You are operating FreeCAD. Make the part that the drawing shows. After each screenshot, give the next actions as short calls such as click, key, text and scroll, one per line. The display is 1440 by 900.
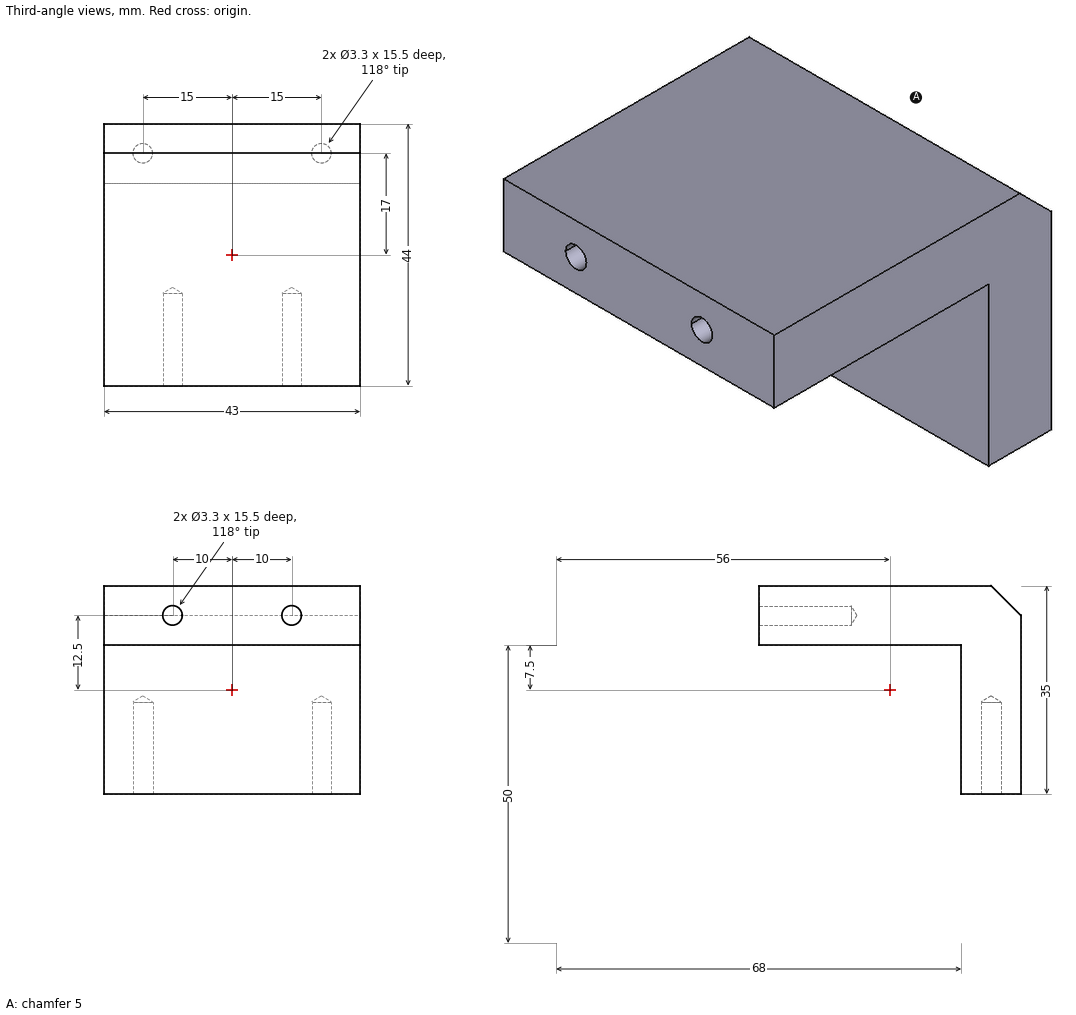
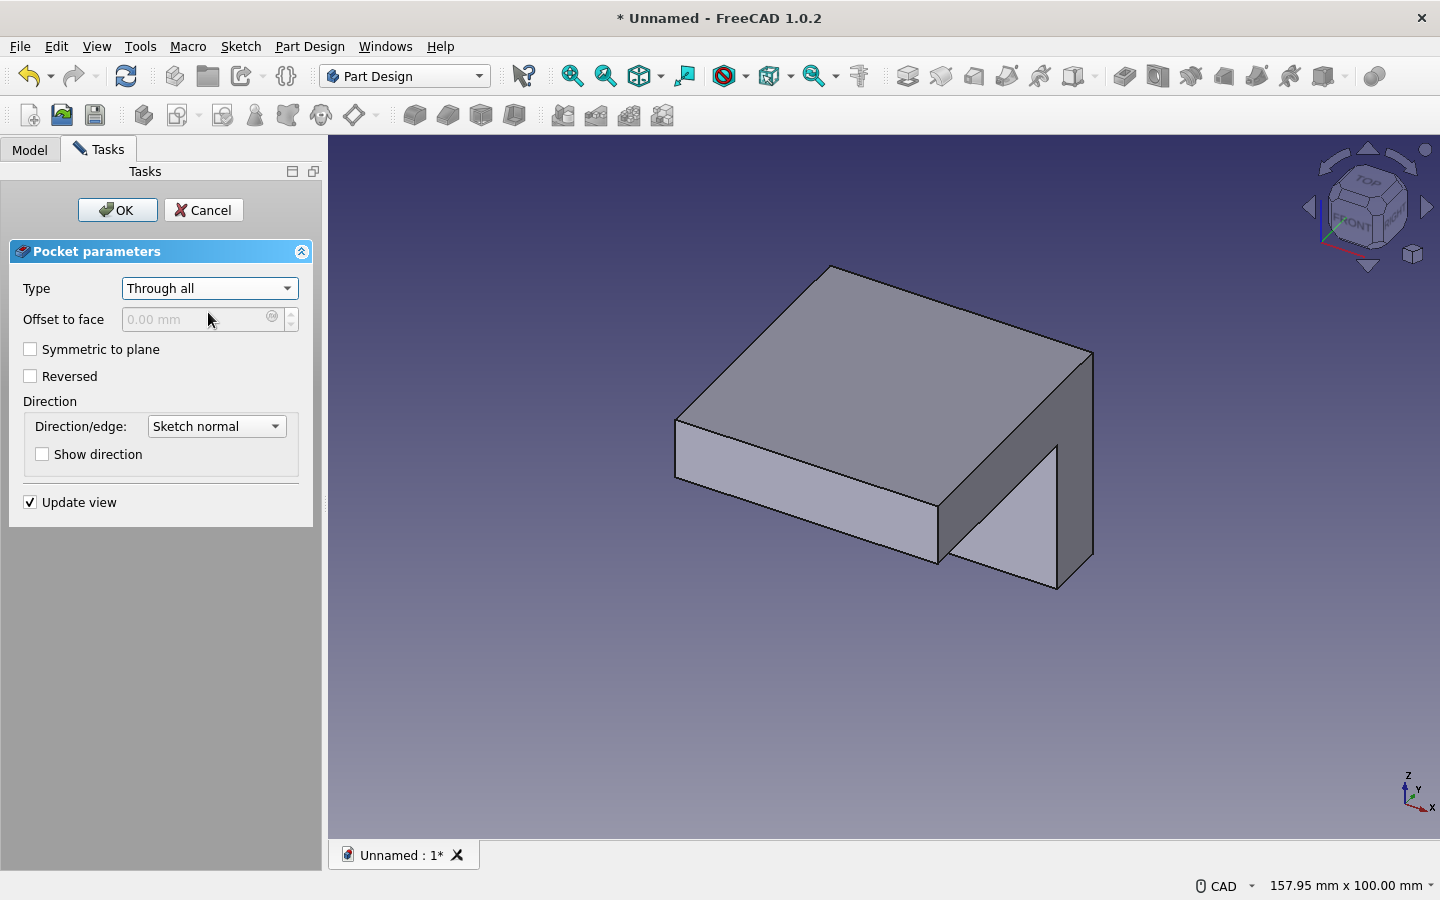
click(118, 210)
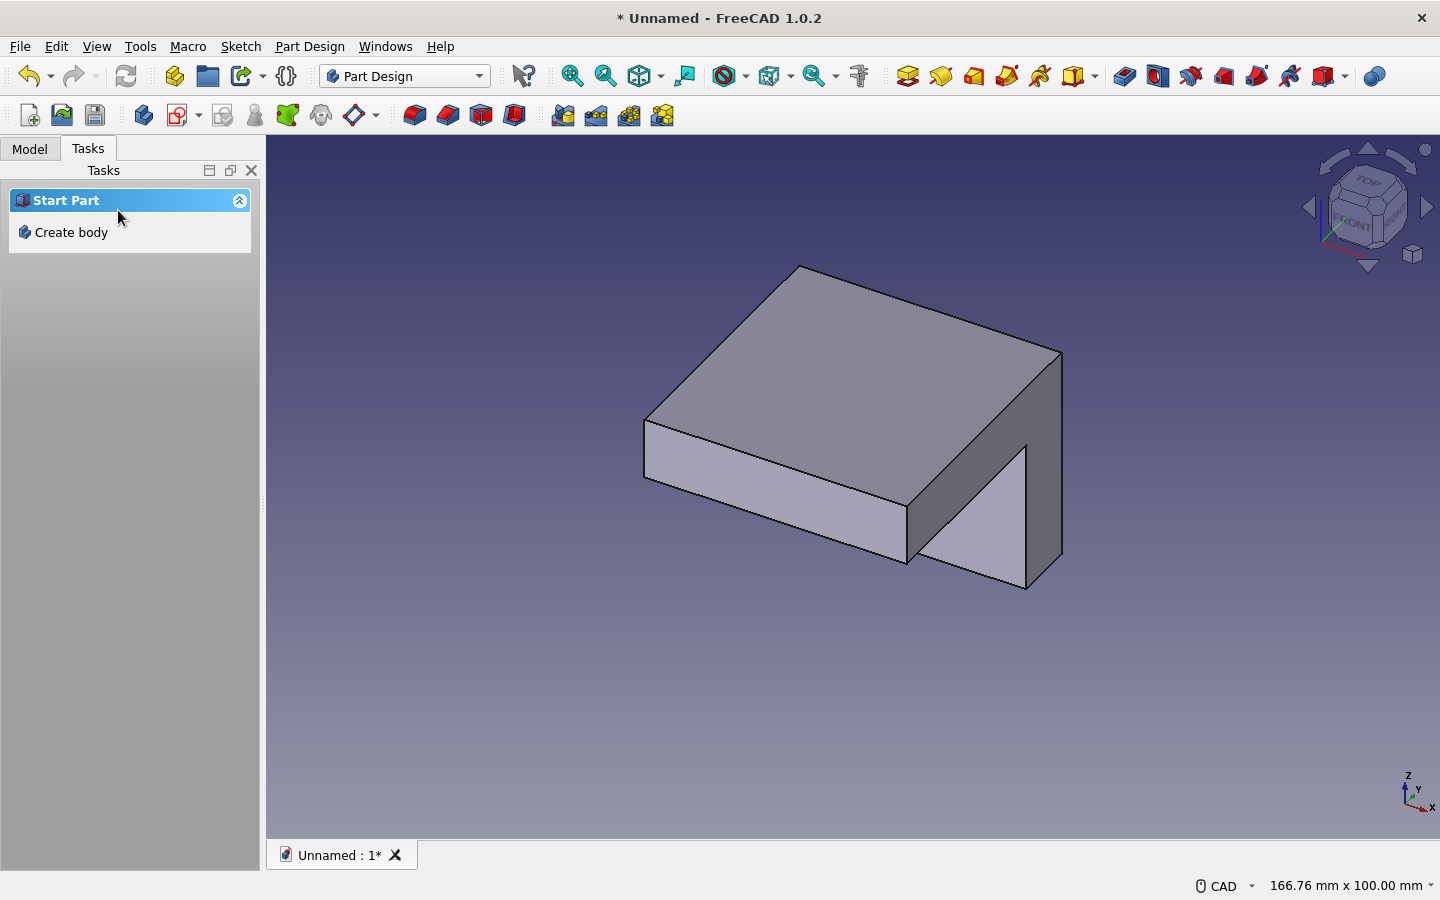
key(5)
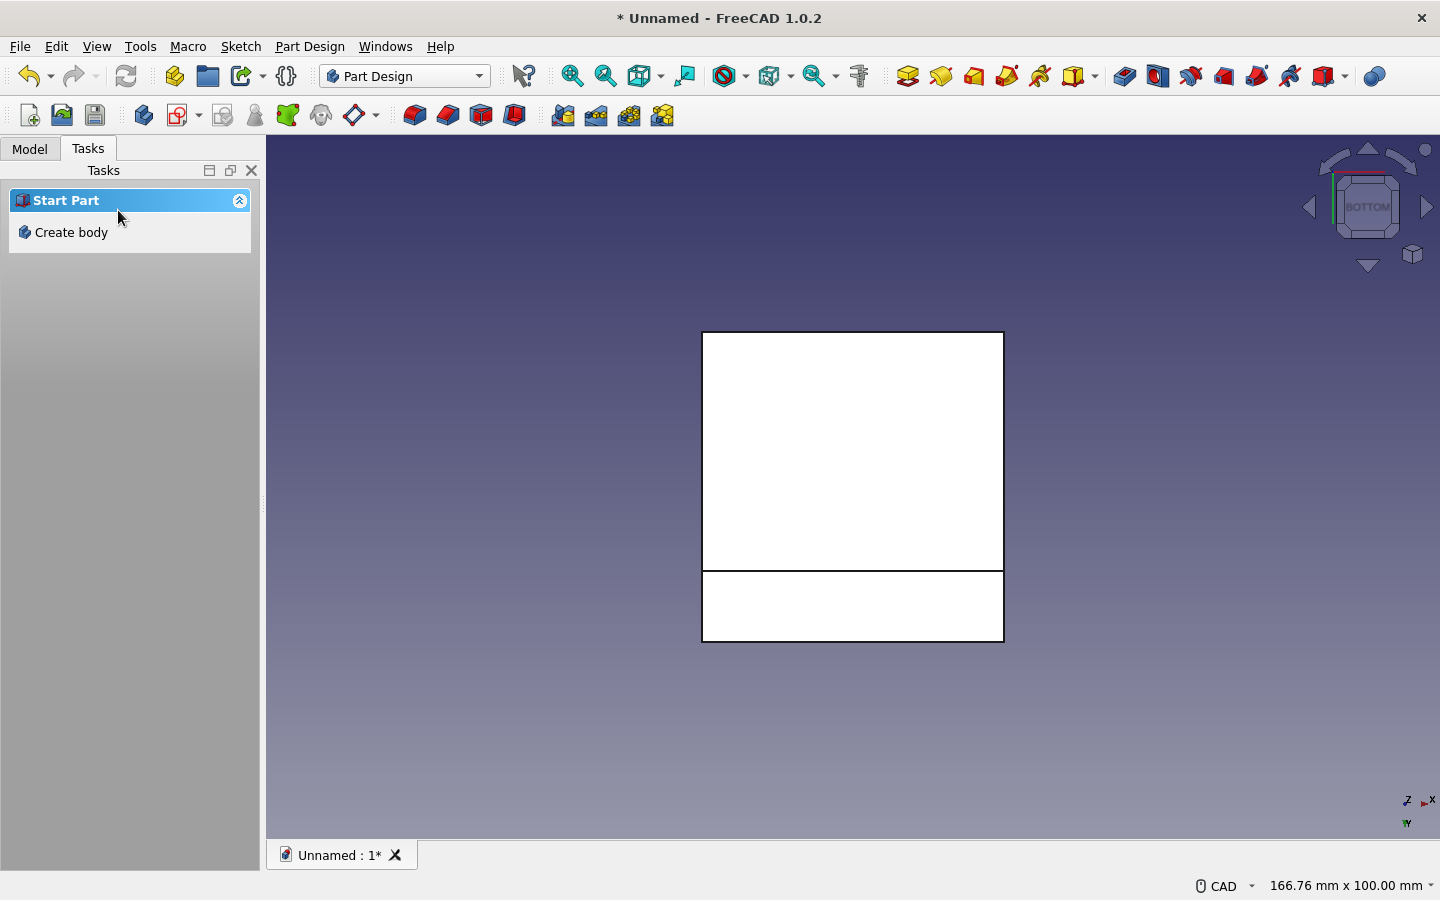
click(573, 76)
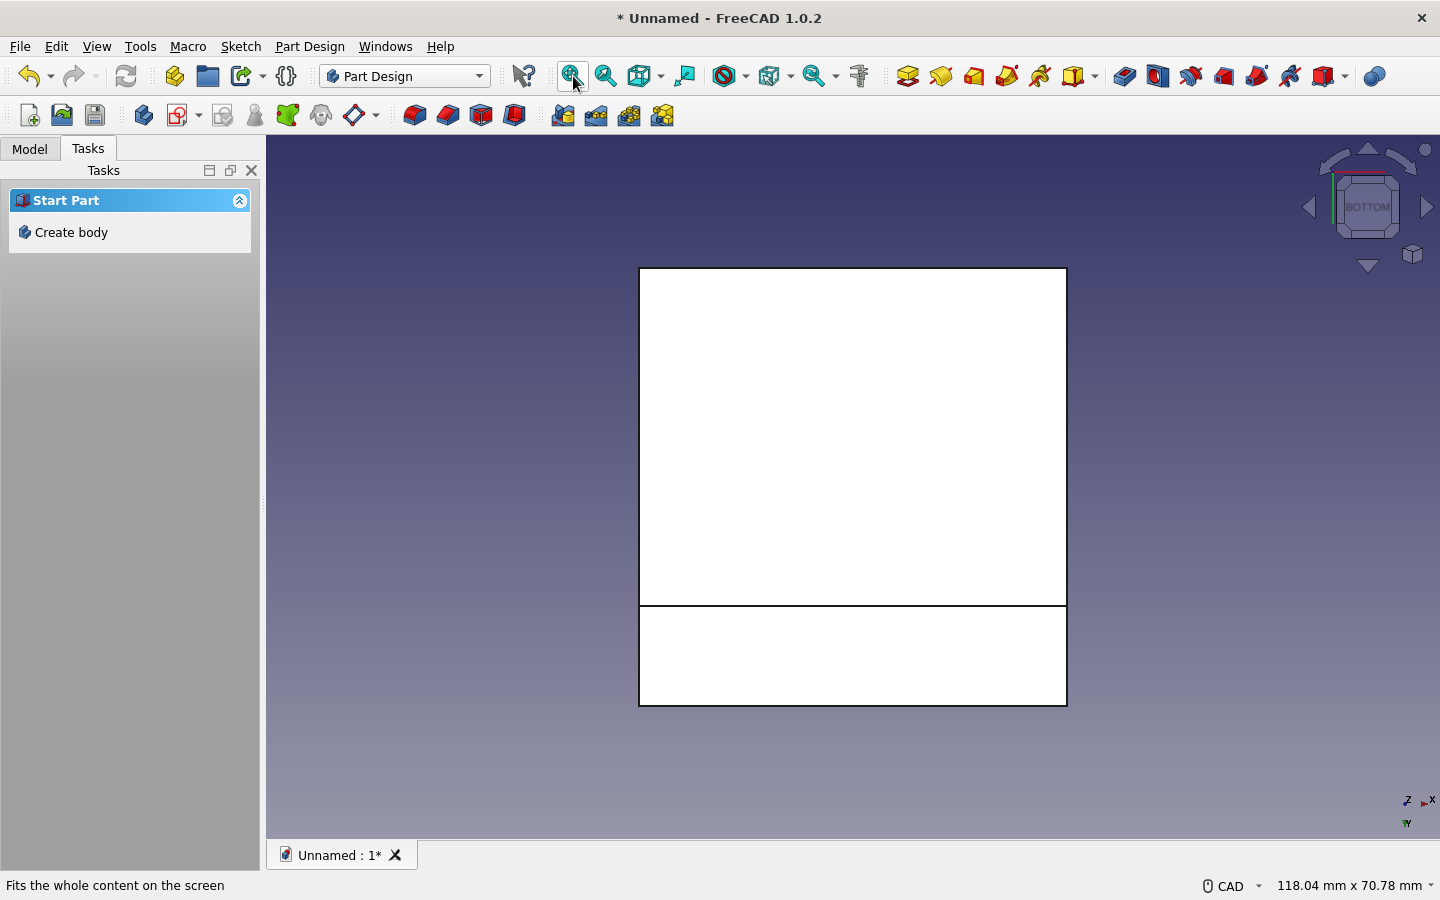
click(975, 655)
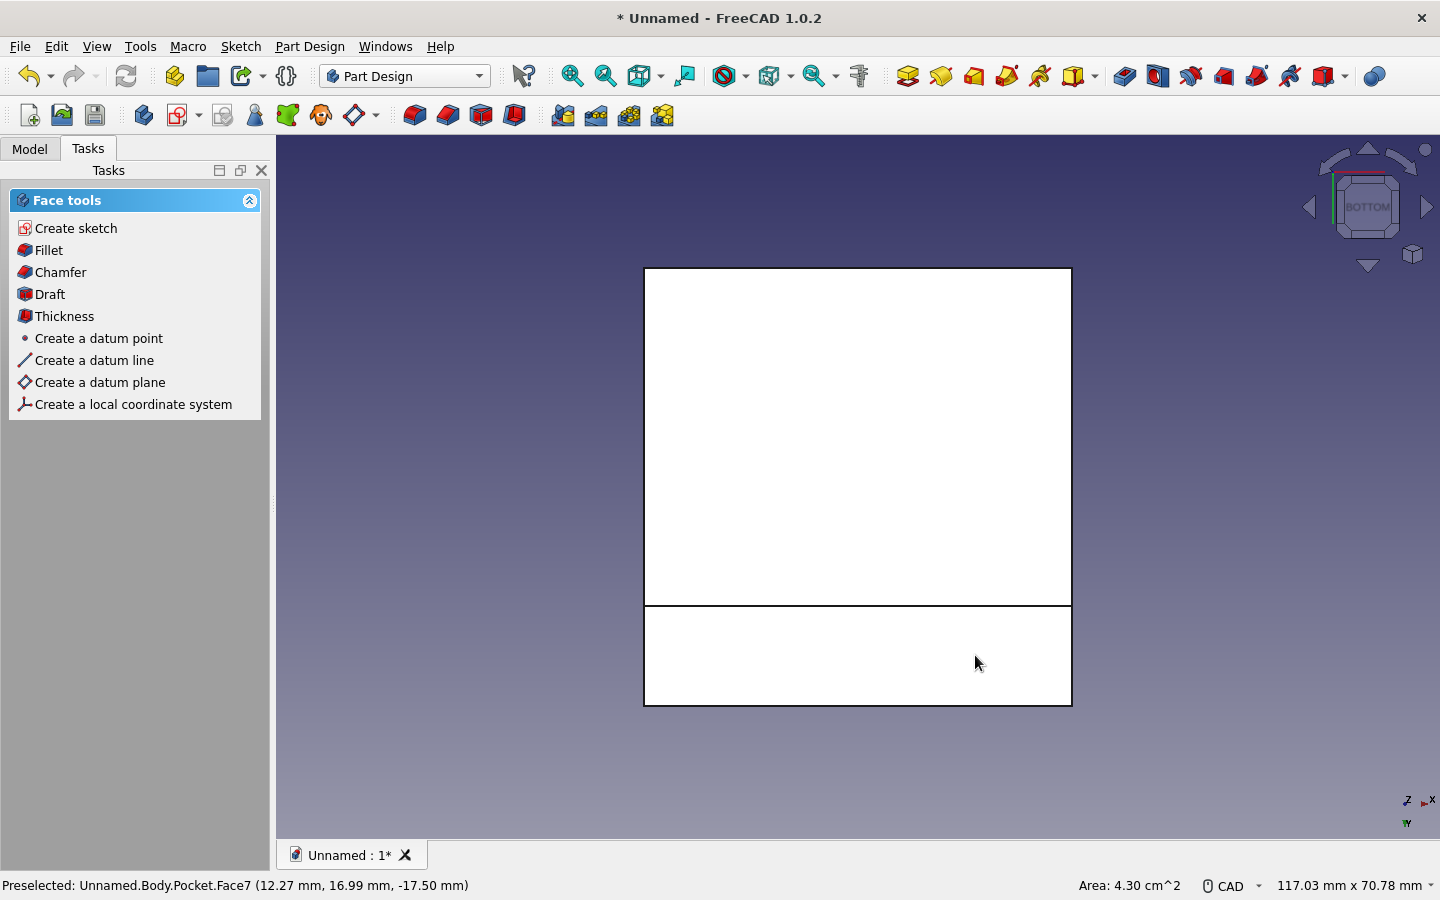
click(176, 116)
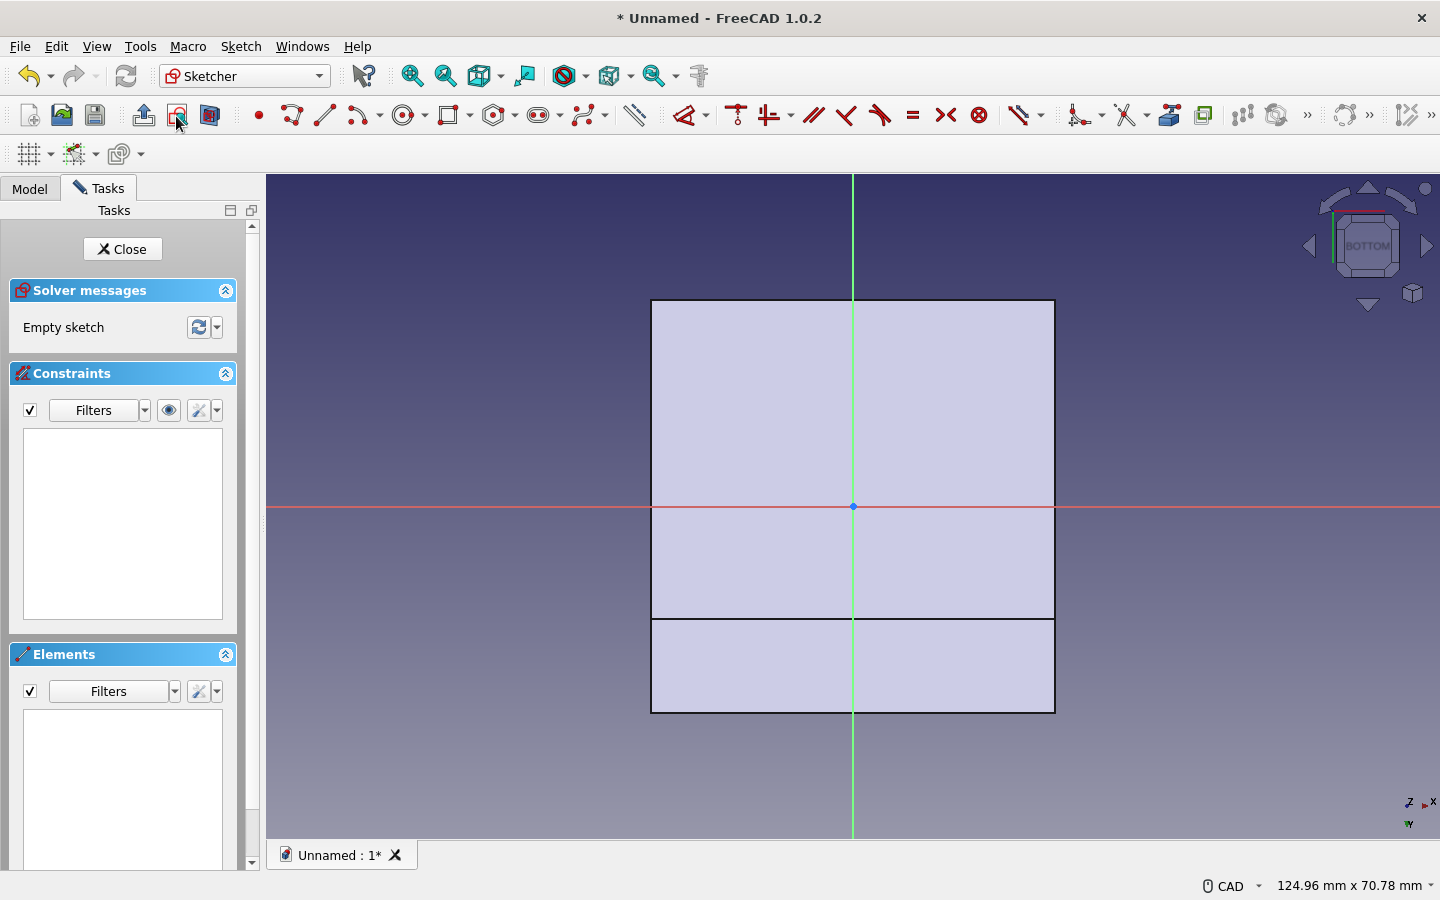
scroll(909, 666, up, 4)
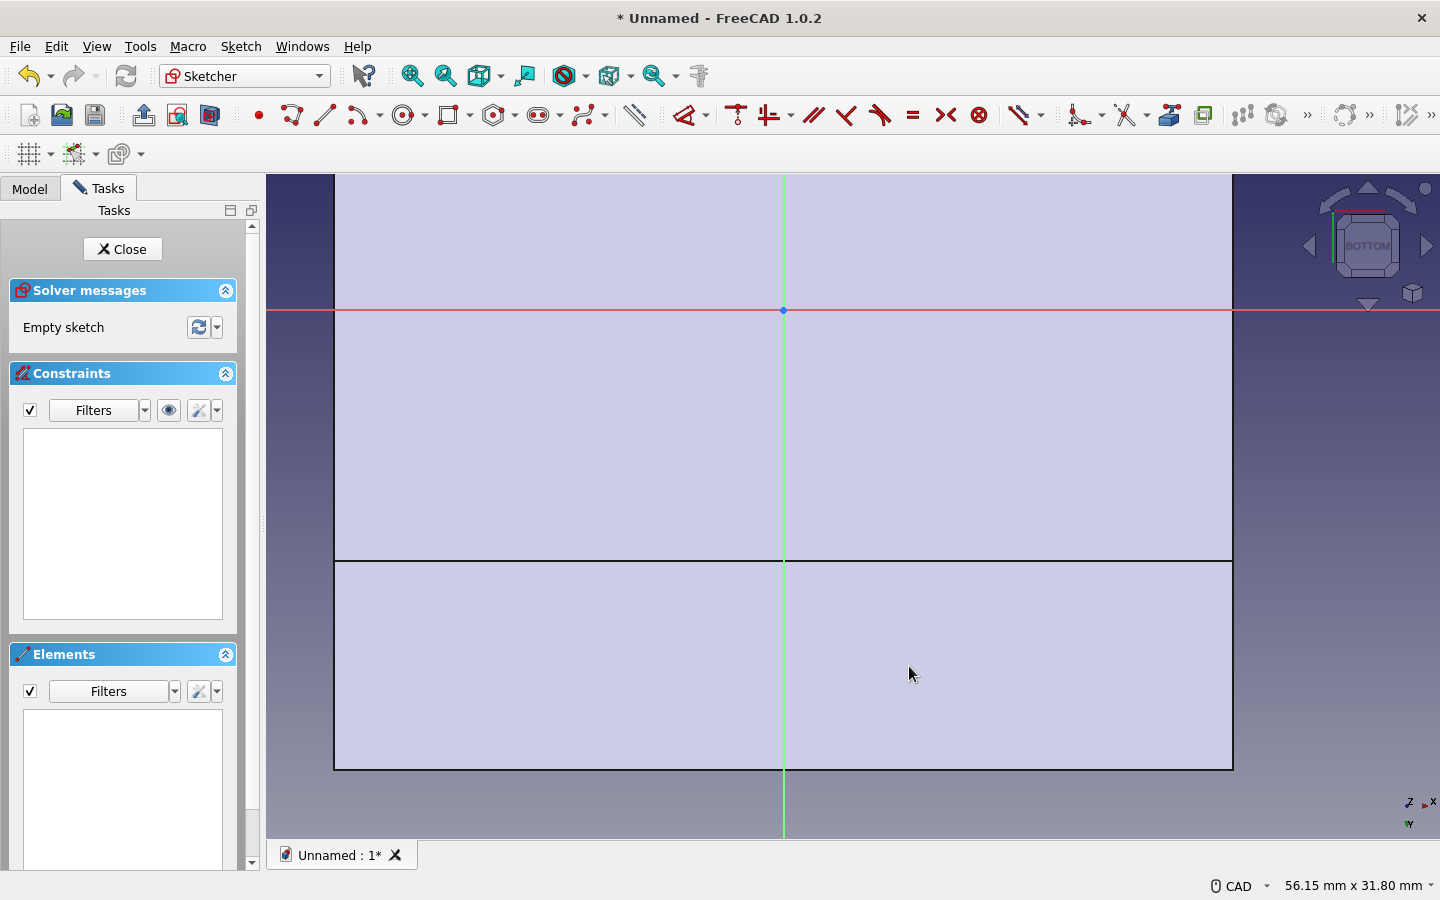
click(402, 116)